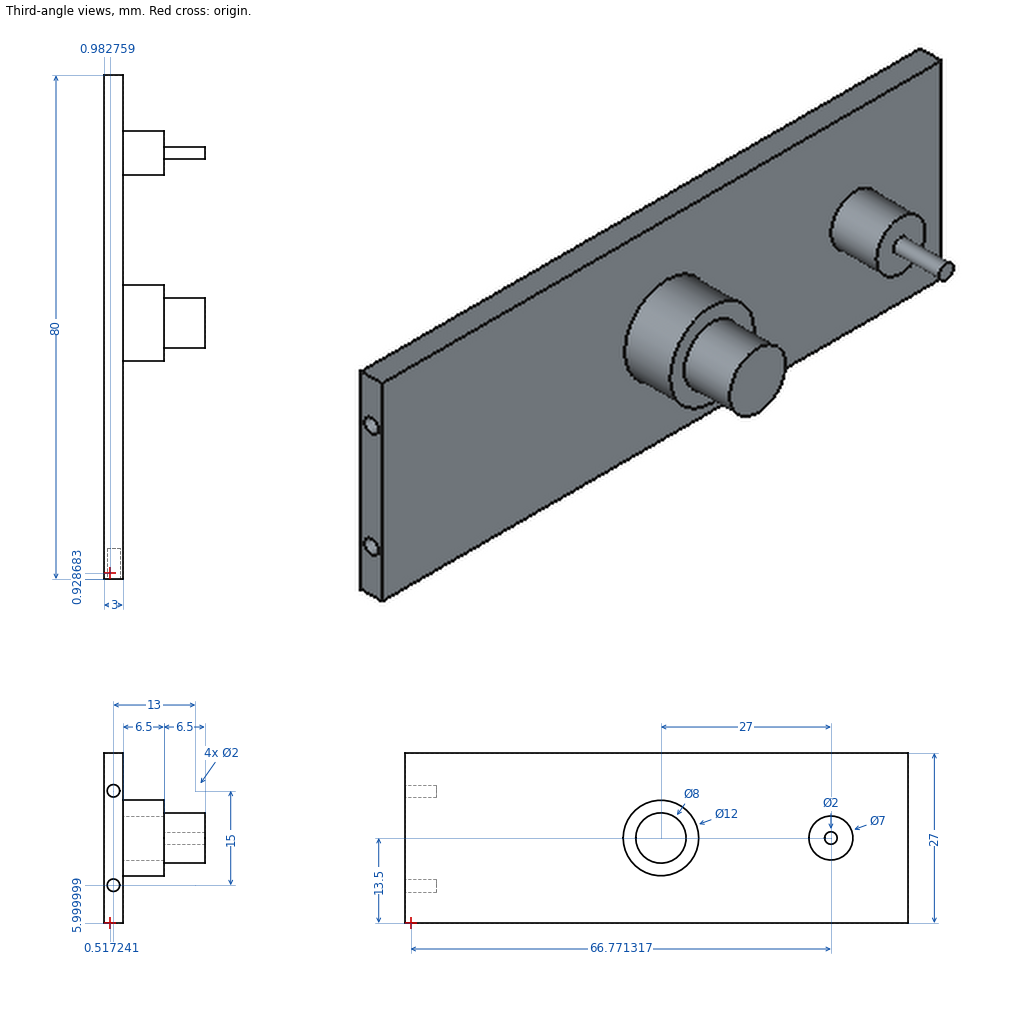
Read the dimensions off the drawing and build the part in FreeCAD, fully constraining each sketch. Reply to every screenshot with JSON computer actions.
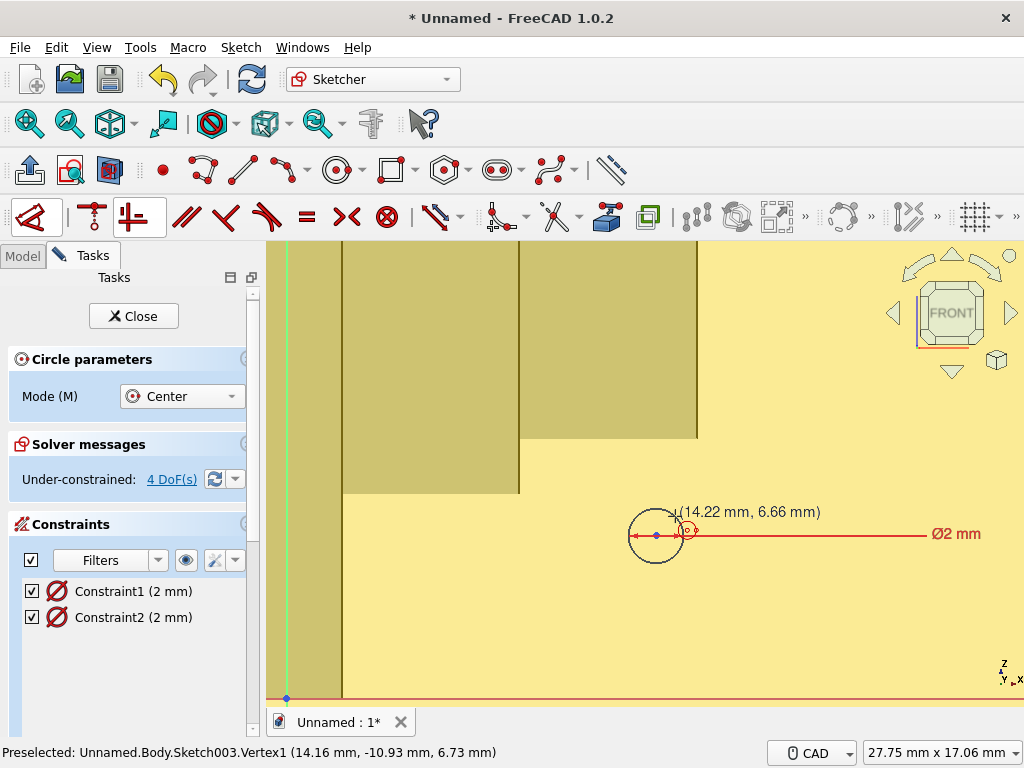
{"action": "scroll", "coordinate": [657, 536], "scroll_direction": "down", "scroll_amount": 4}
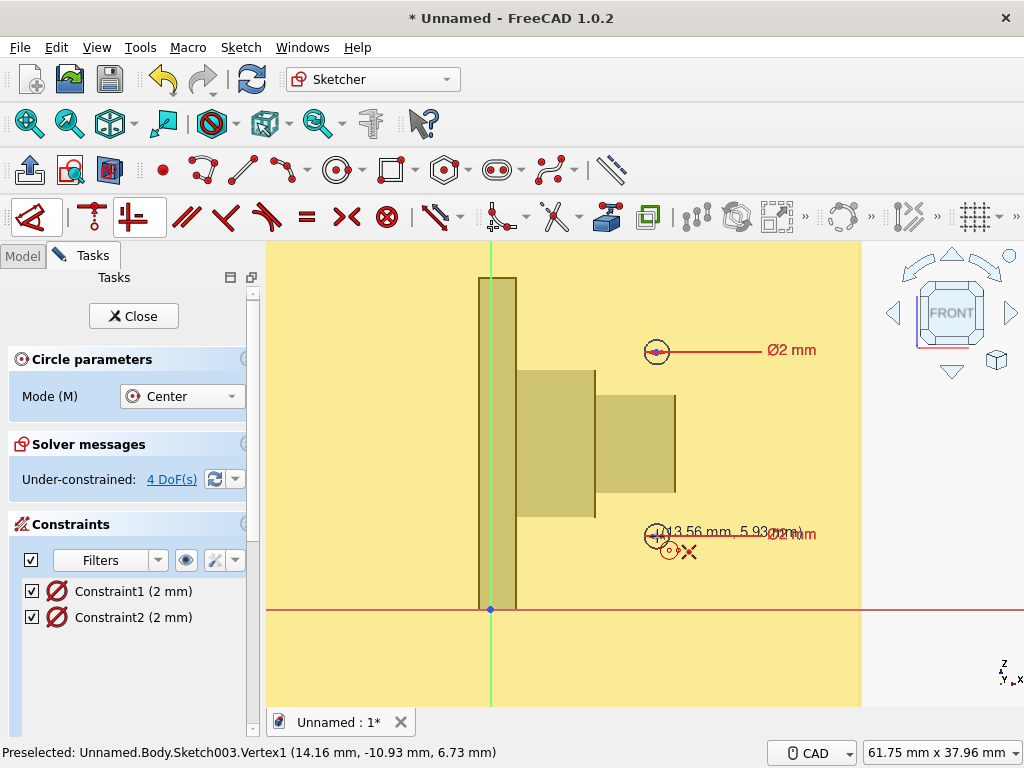
{"action": "scroll", "coordinate": [497, 352], "scroll_direction": "up", "scroll_amount": 5}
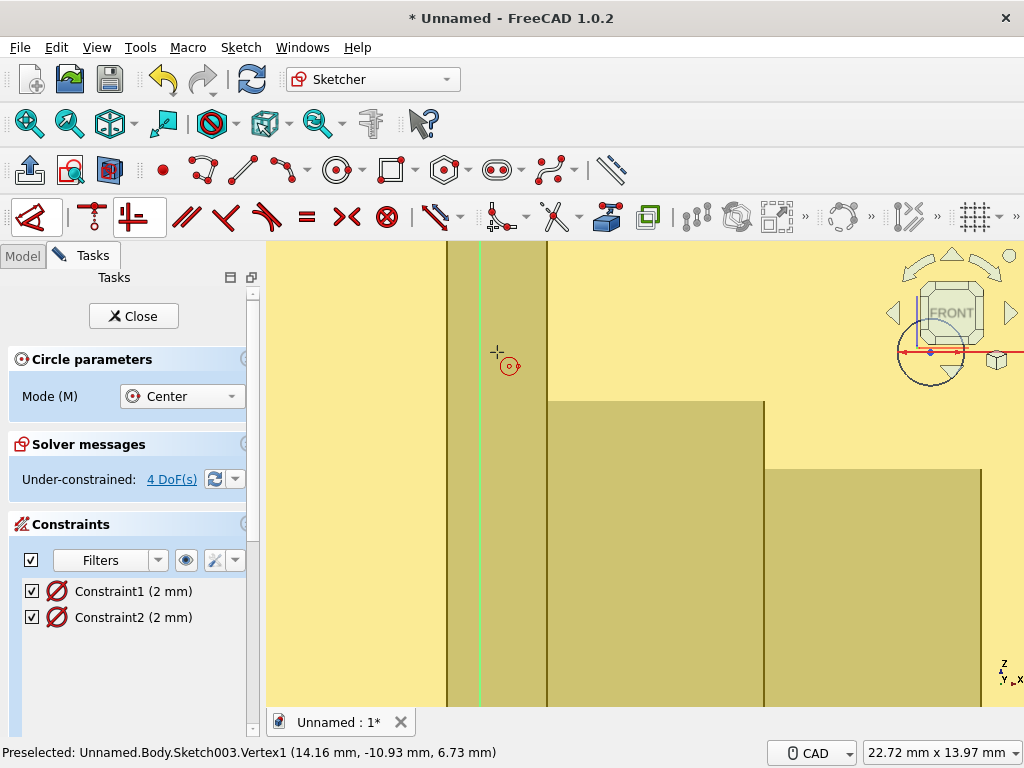
{"action": "left_click", "coordinate": [497, 351]}
{"action": "mouse_move", "coordinate": [521, 327]}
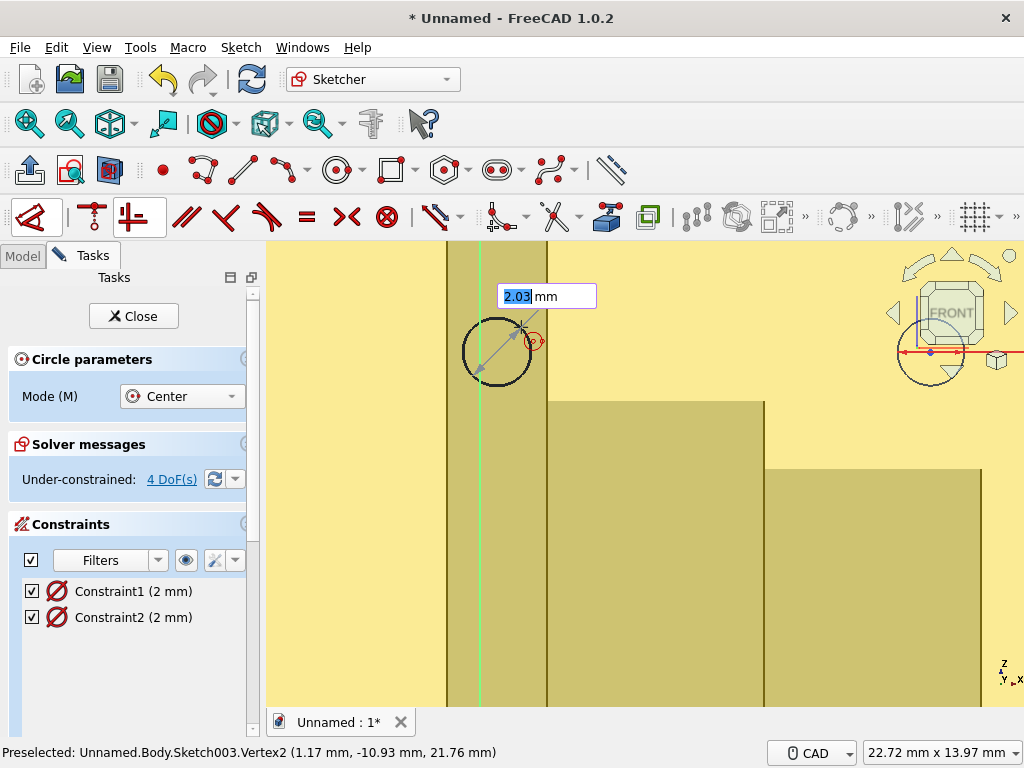
{"action": "type", "text": "2"}
{"action": "key", "text": "Return"}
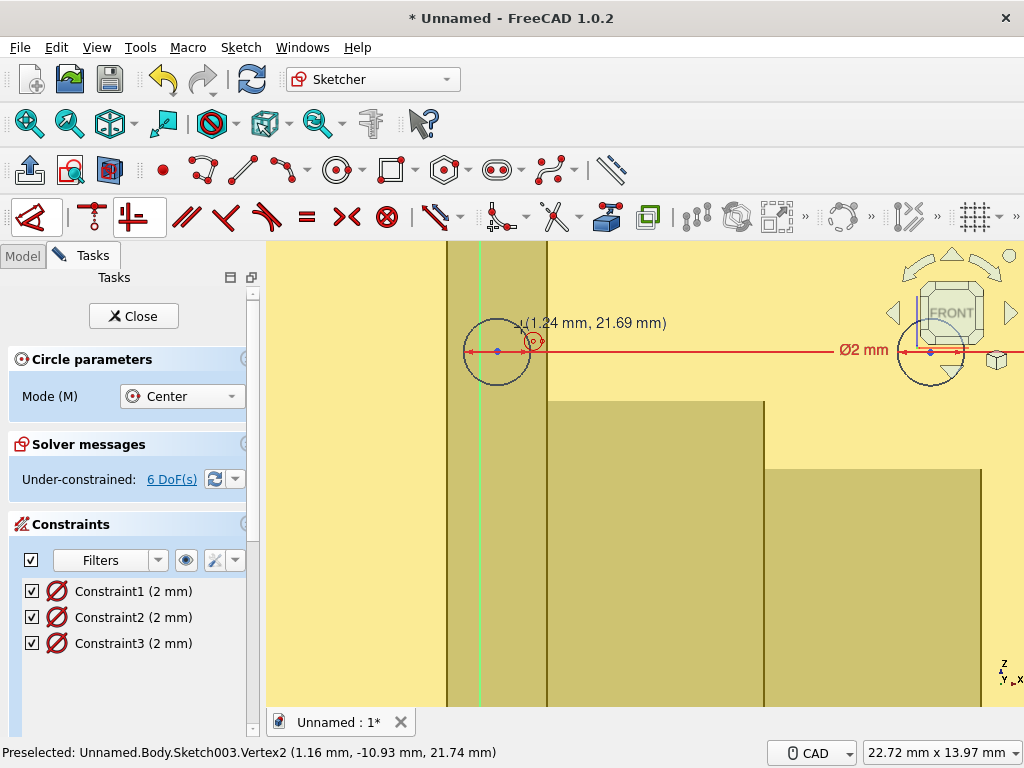
{"action": "scroll", "coordinate": [497, 351], "scroll_direction": "down", "scroll_amount": 5}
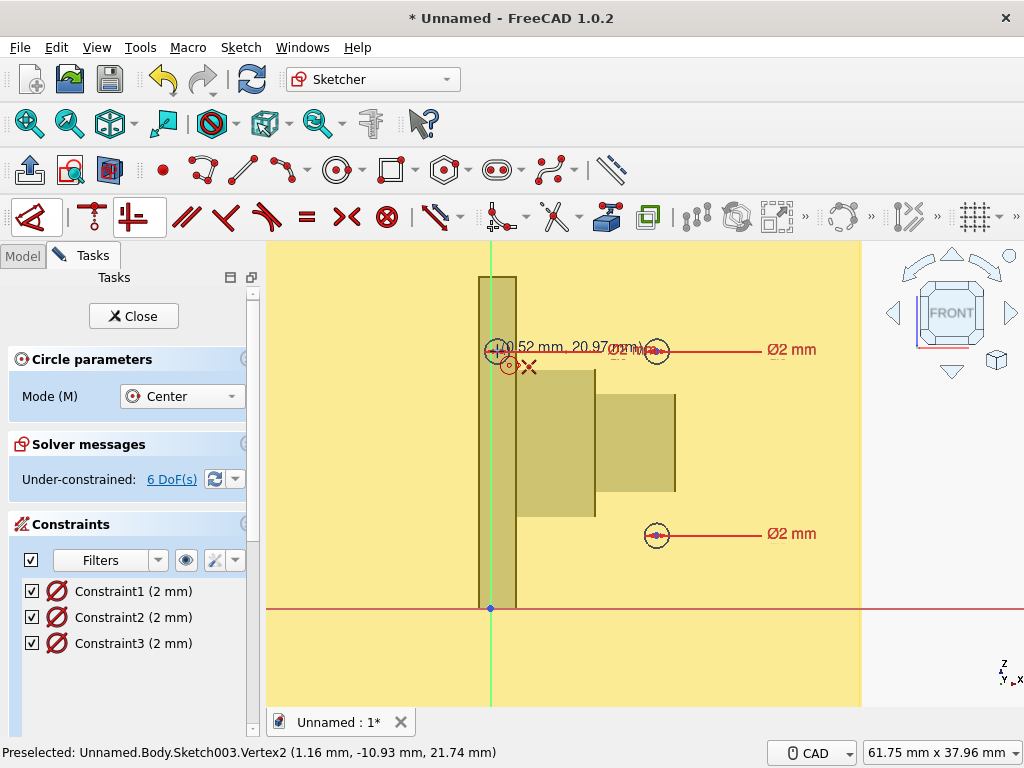
{"action": "scroll", "coordinate": [497, 535], "scroll_direction": "up", "scroll_amount": 5}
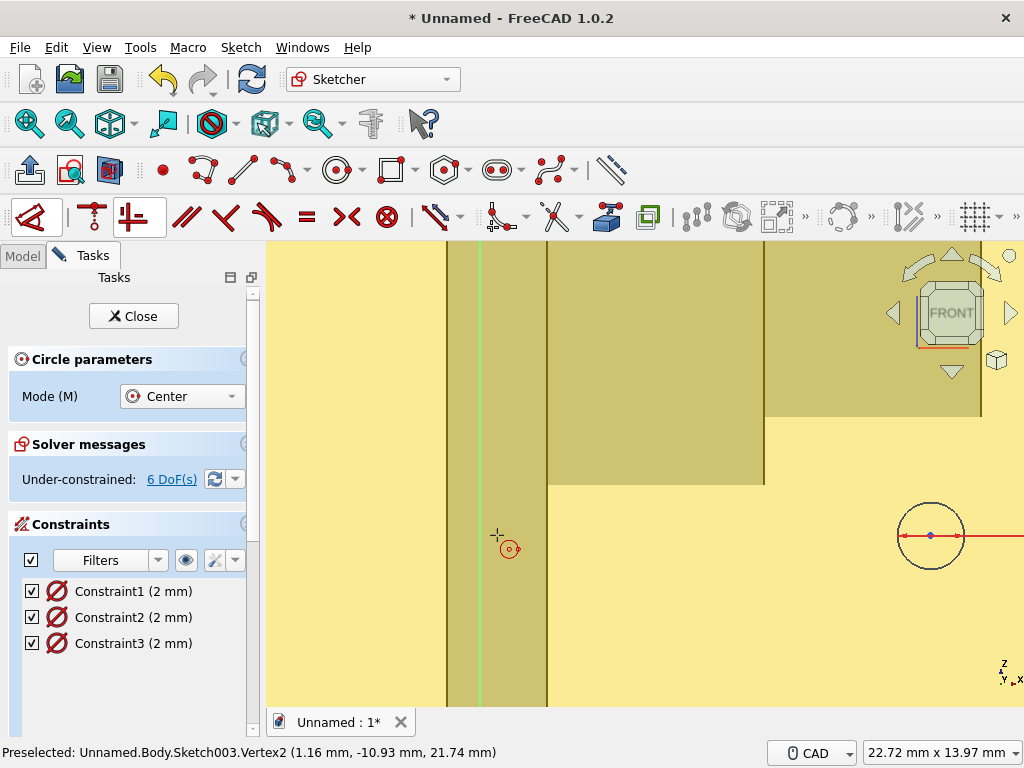
{"action": "left_click", "coordinate": [497, 535]}
{"action": "mouse_move", "coordinate": [521, 511]}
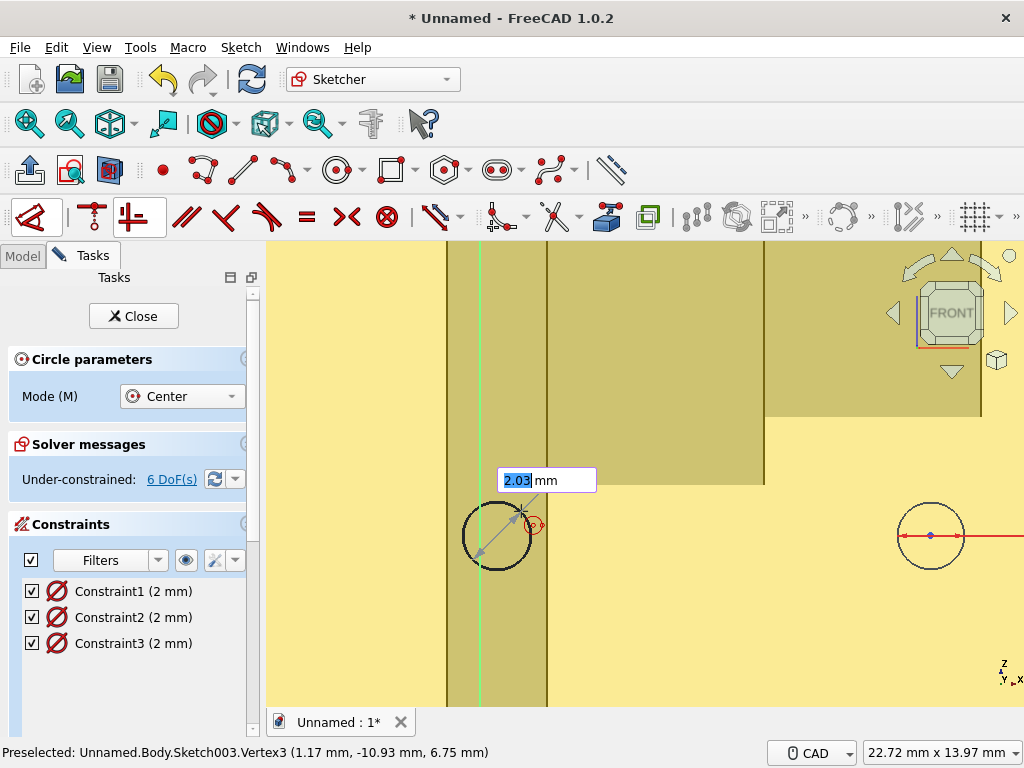
{"action": "type", "text": "2"}
{"action": "key", "text": "Return"}
{"action": "key", "text": "Escape"}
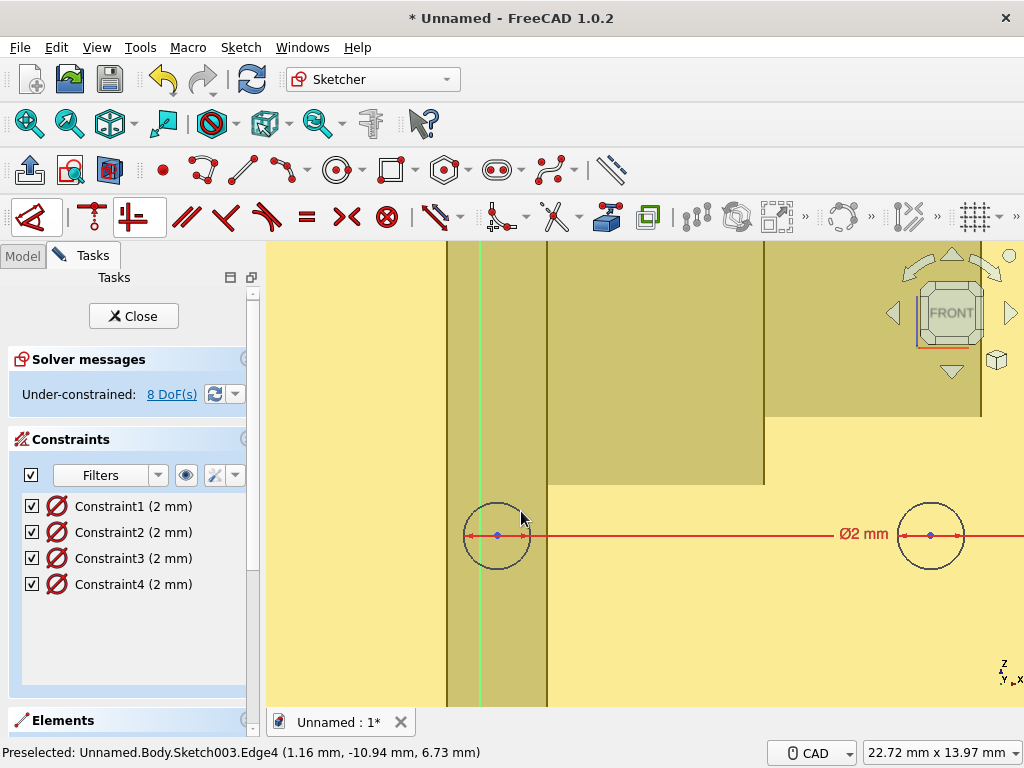
{"action": "scroll", "coordinate": [497, 536], "scroll_direction": "down", "scroll_amount": 5}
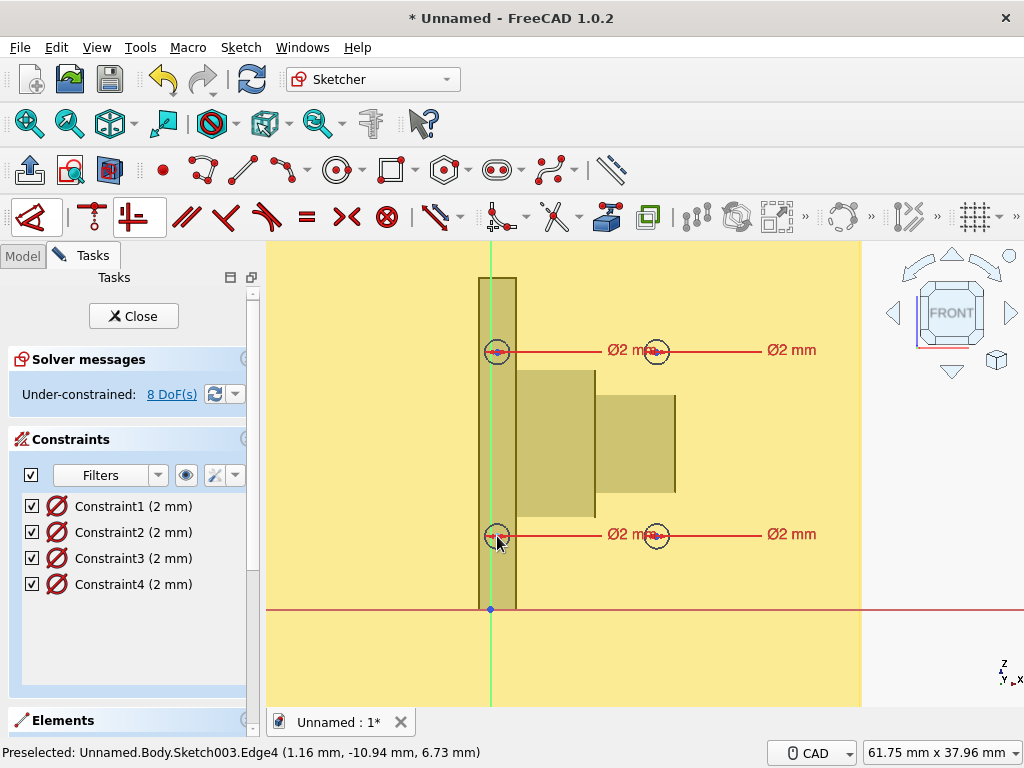
{"action": "left_click", "coordinate": [657, 352]}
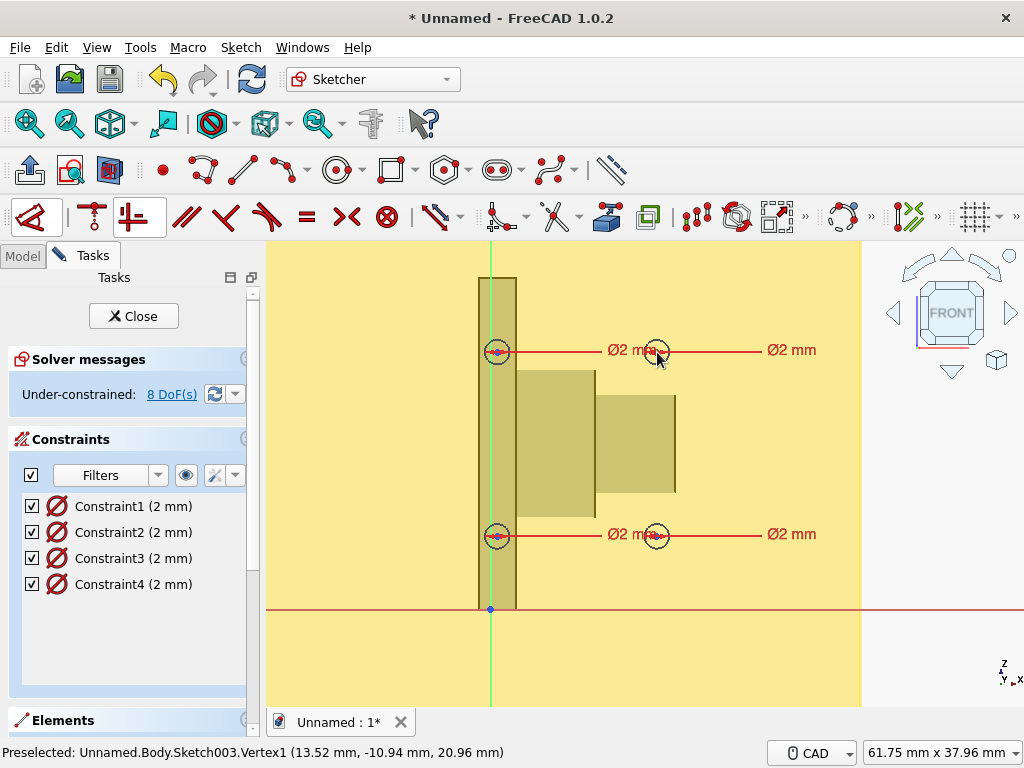
{"action": "left_click", "coordinate": [657, 536]}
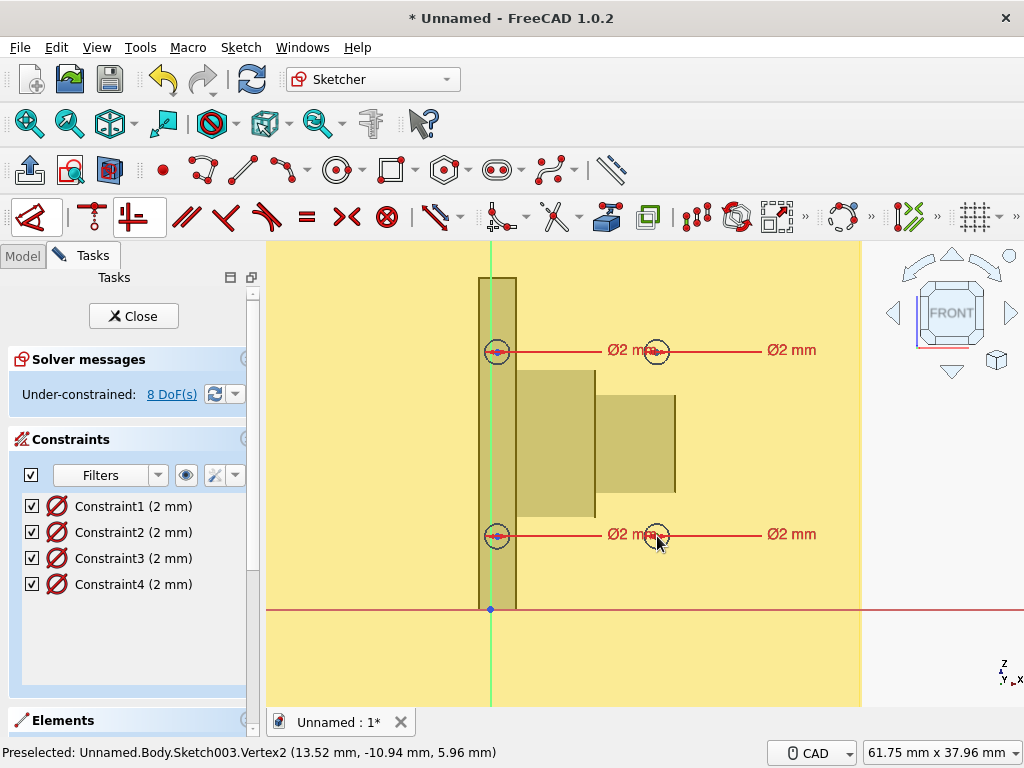
{"action": "left_click", "coordinate": [160, 218]}